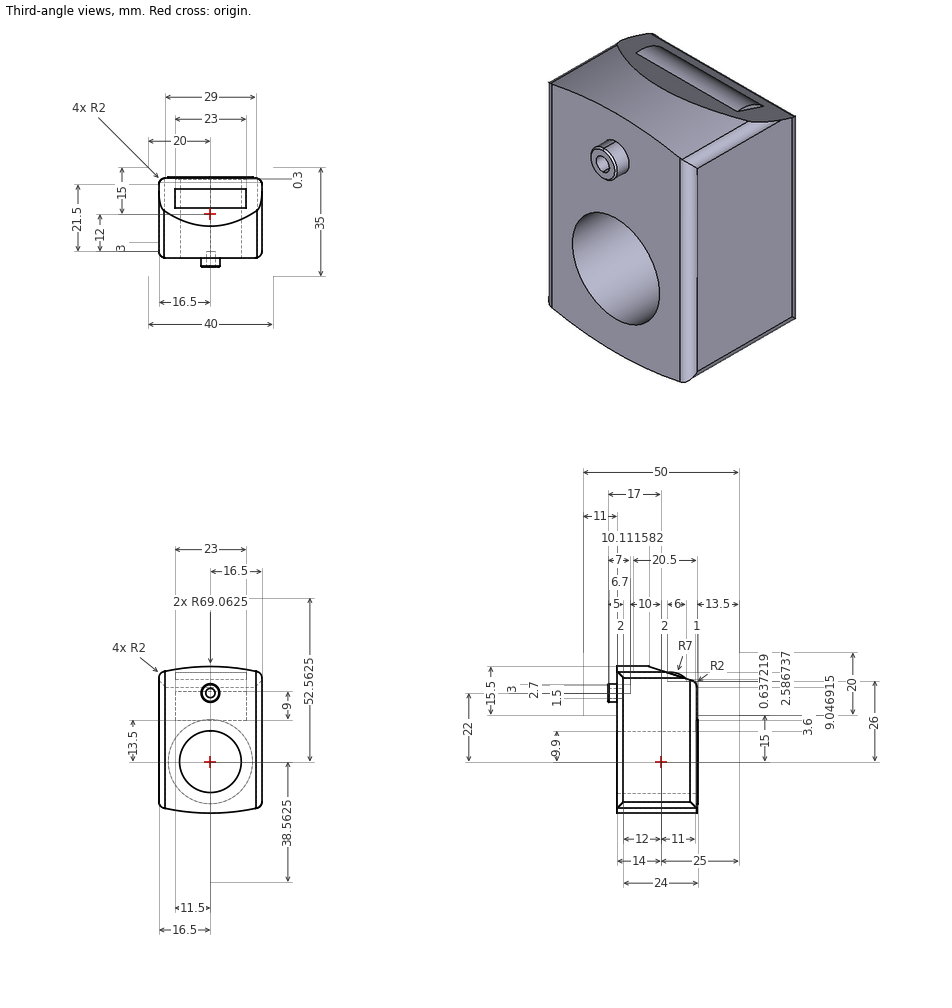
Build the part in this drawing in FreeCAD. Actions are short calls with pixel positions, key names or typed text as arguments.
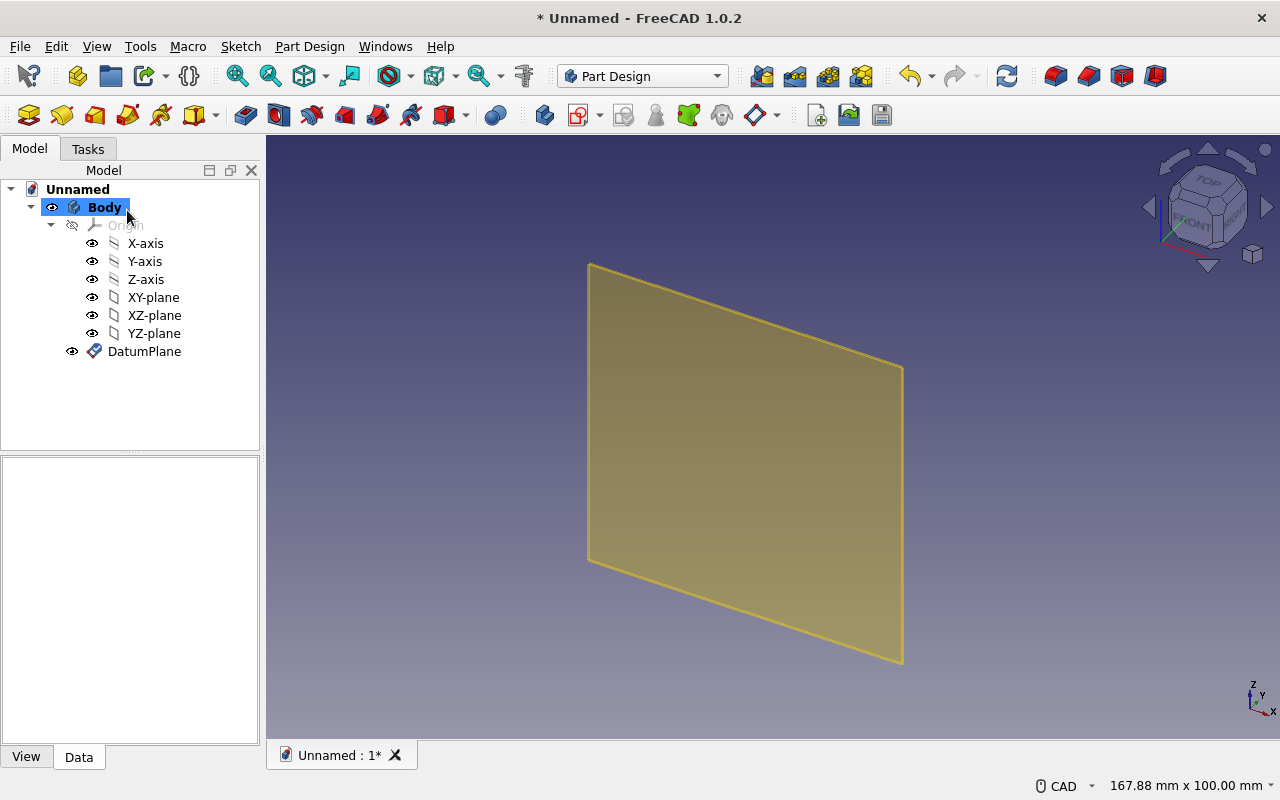
click(117, 351)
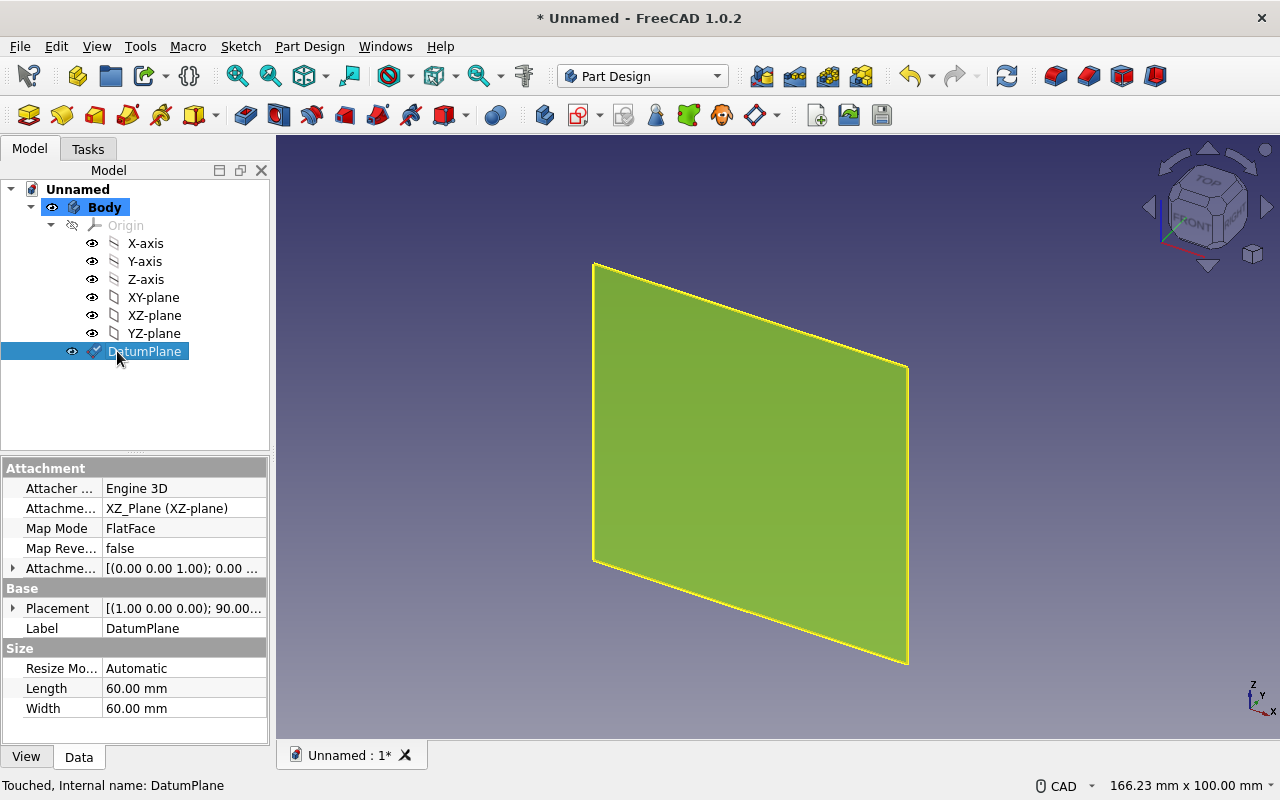
click(578, 116)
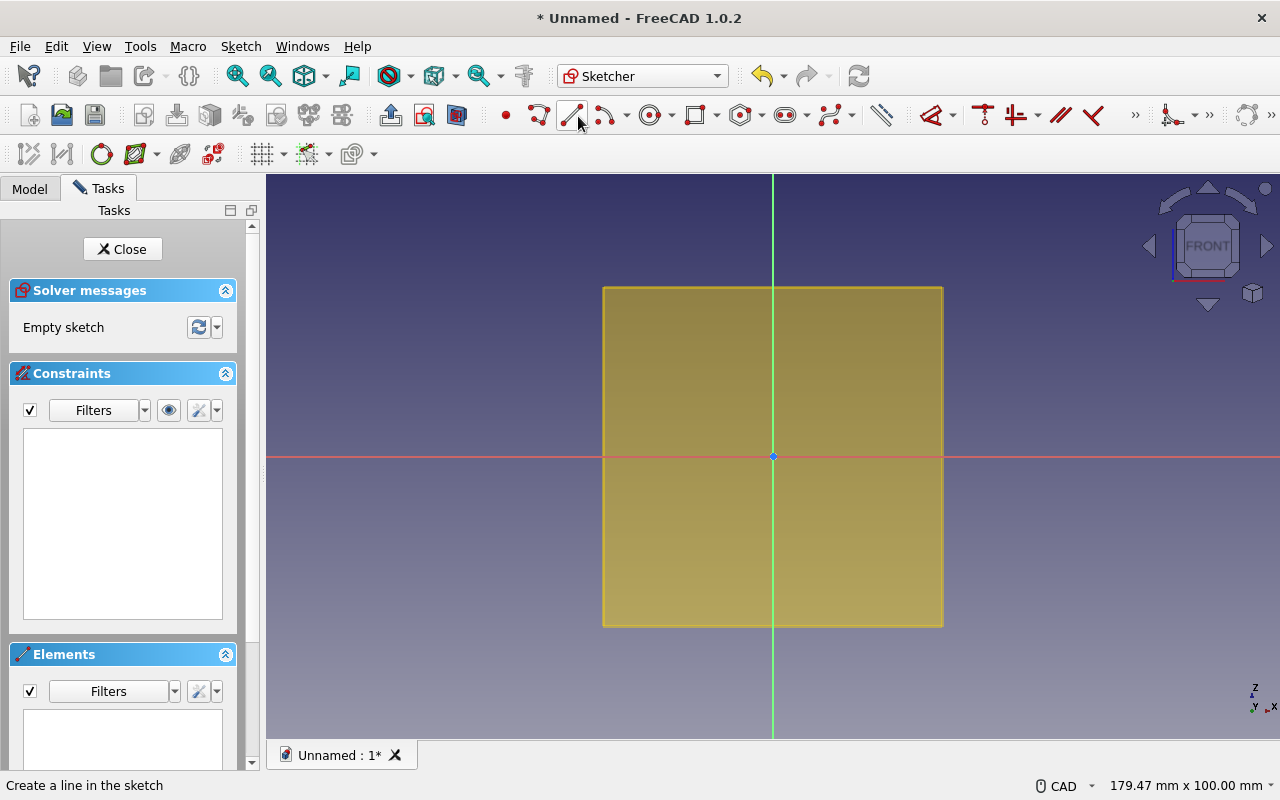
scroll(912, 337, up, 2)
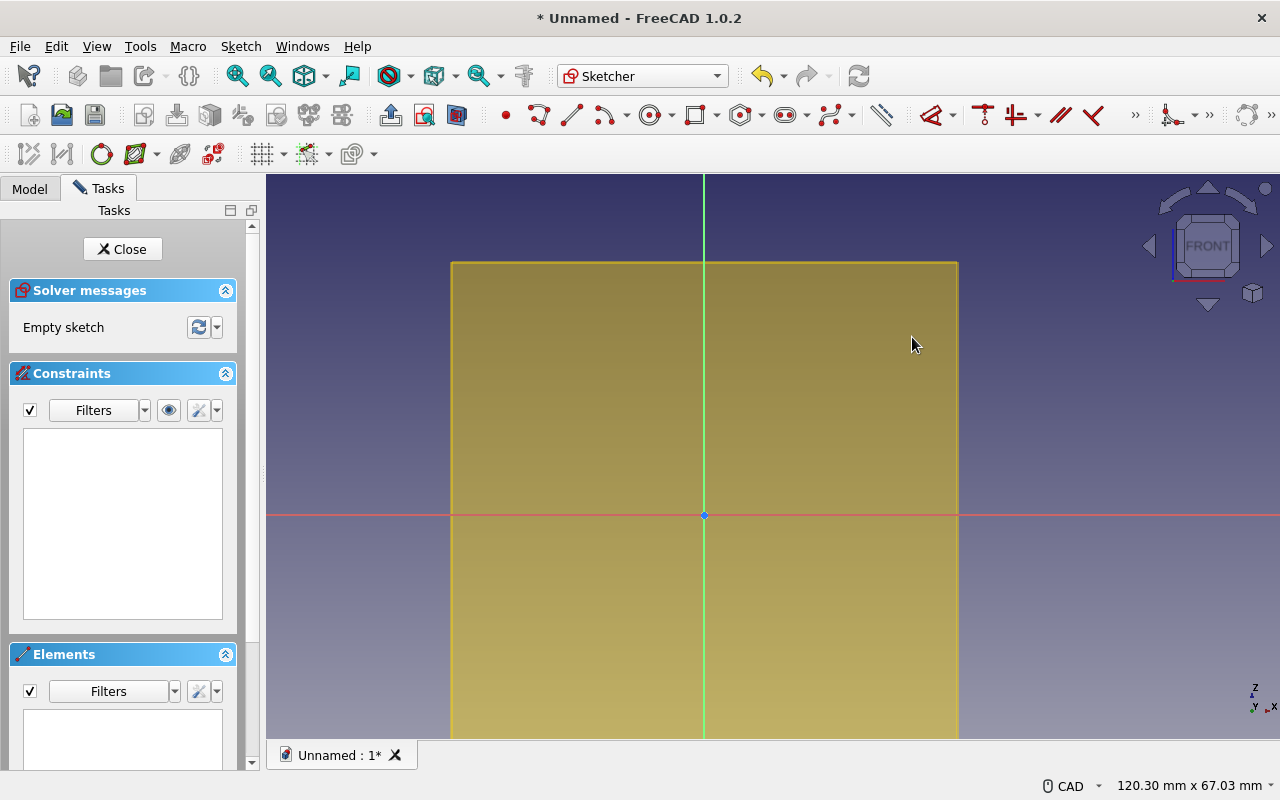
click(572, 116)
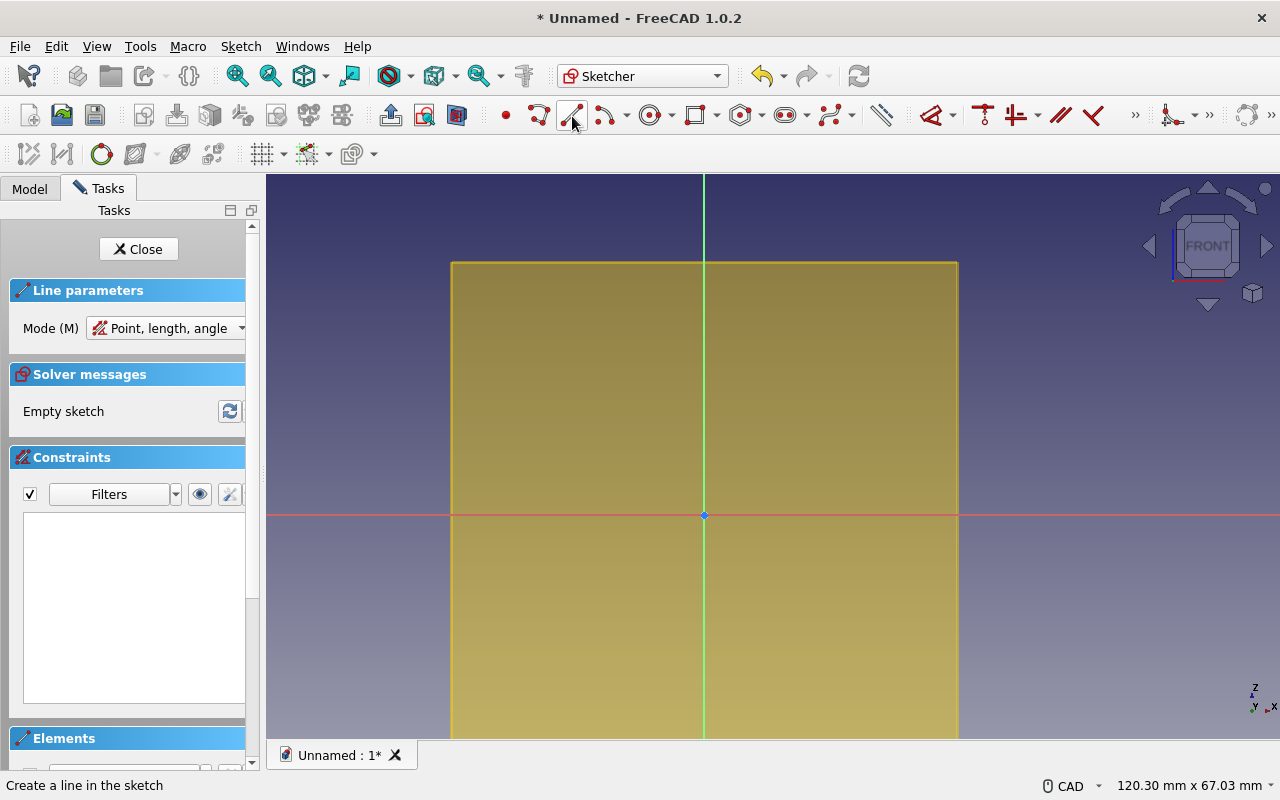
click(565, 624)
click(565, 288)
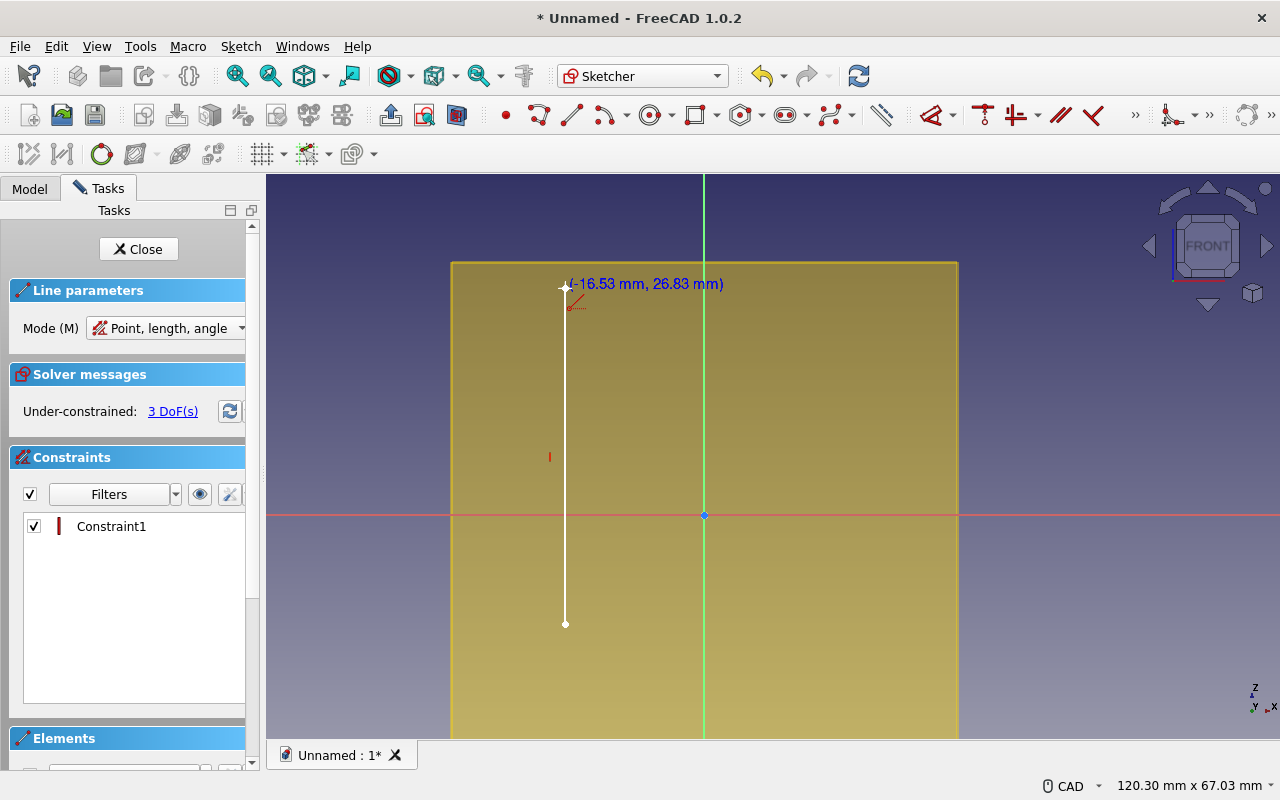
click(843, 288)
click(843, 624)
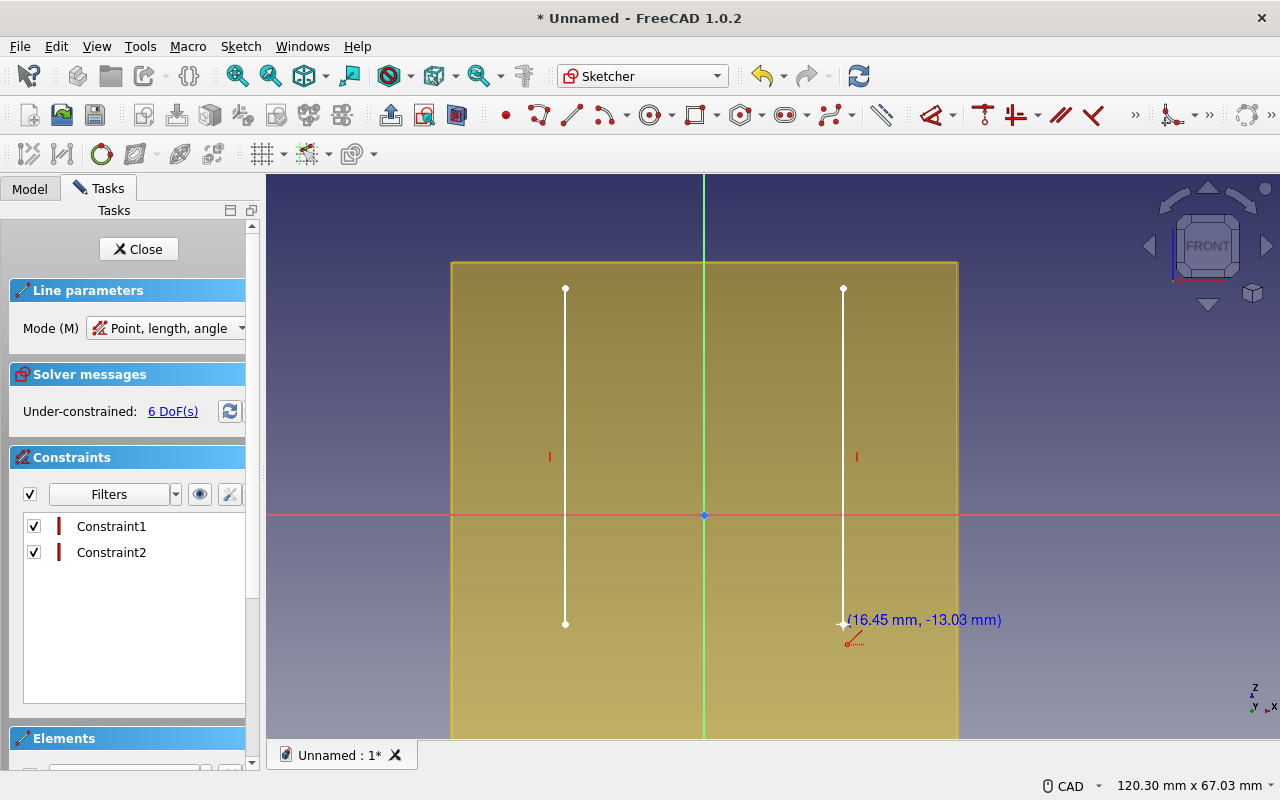
key(g)
key(3)
key(a)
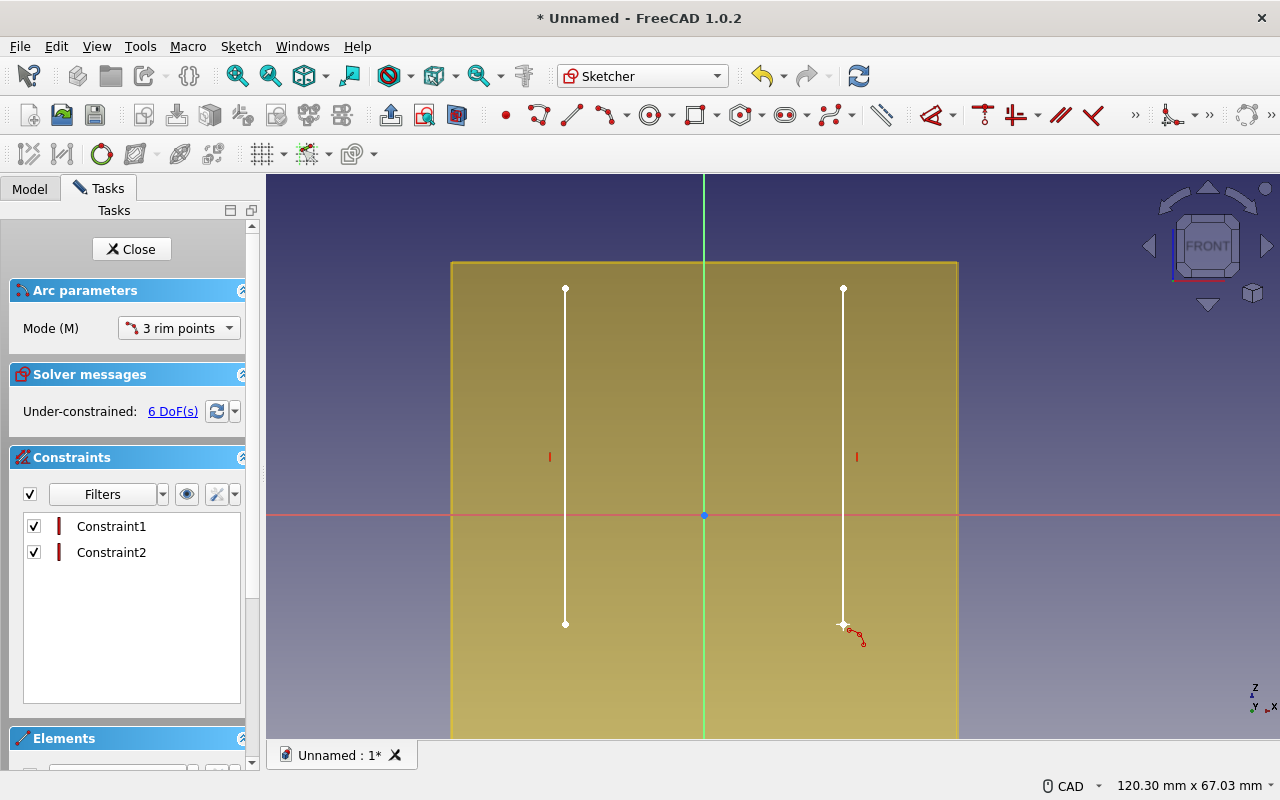
click(565, 289)
click(578, 272)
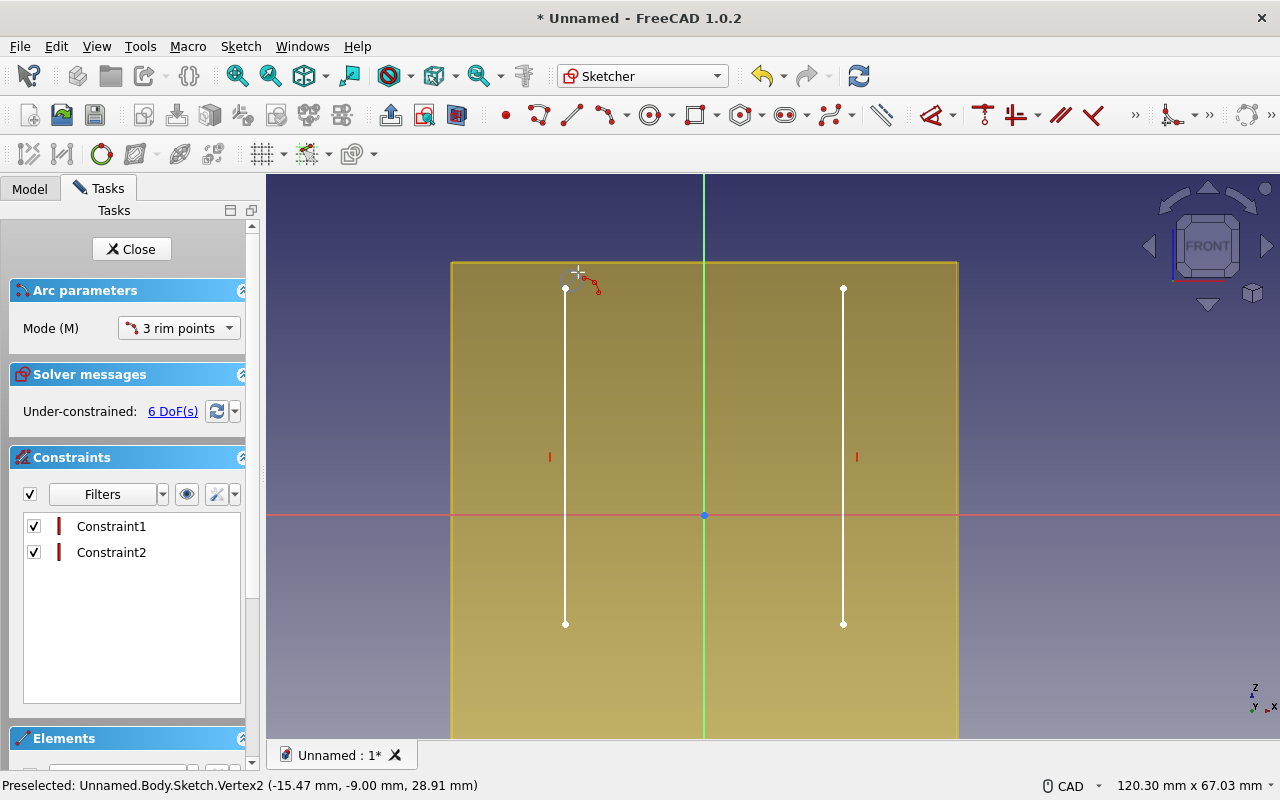
scroll(569, 278, up, 8)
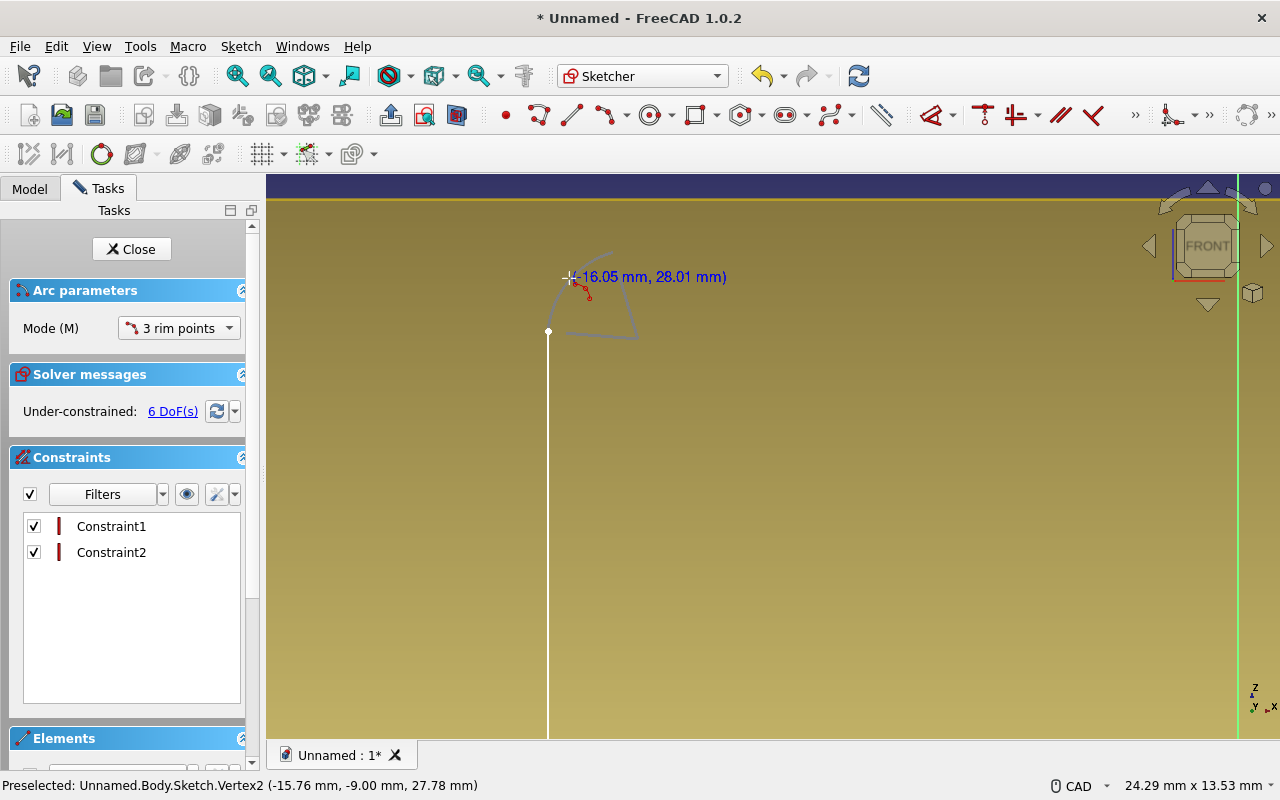
click(568, 276)